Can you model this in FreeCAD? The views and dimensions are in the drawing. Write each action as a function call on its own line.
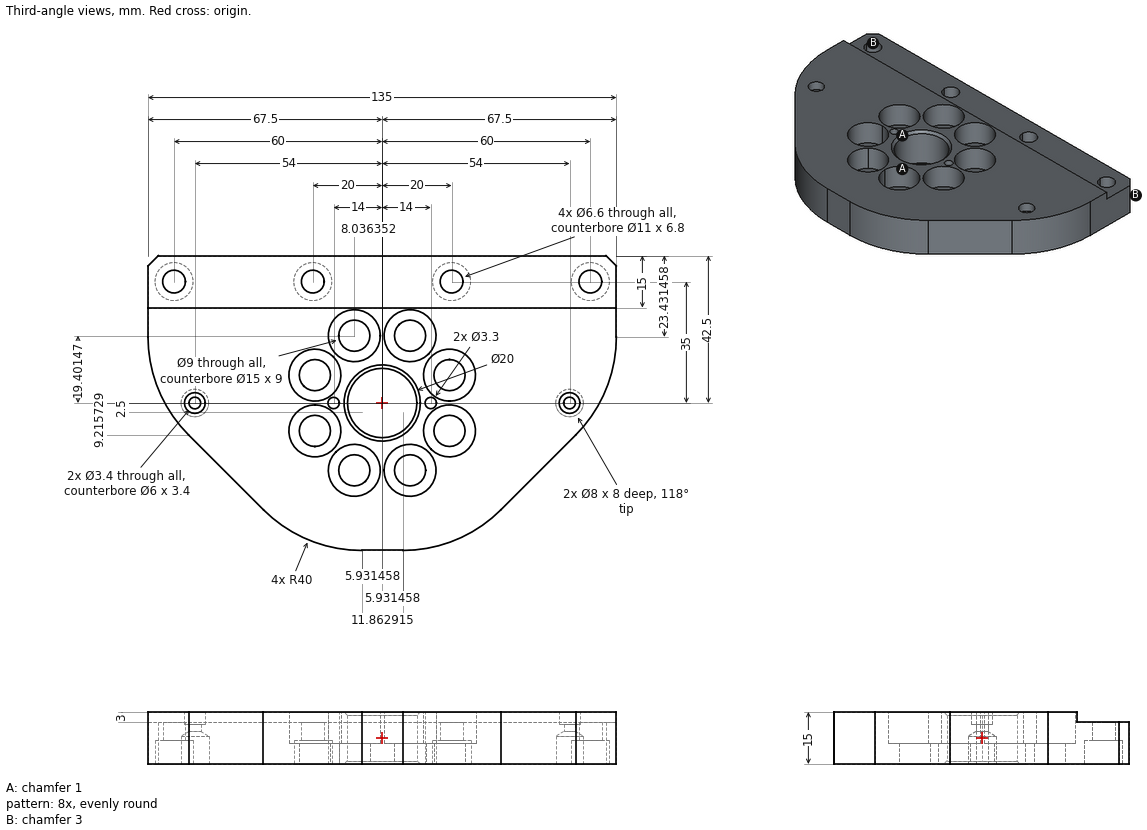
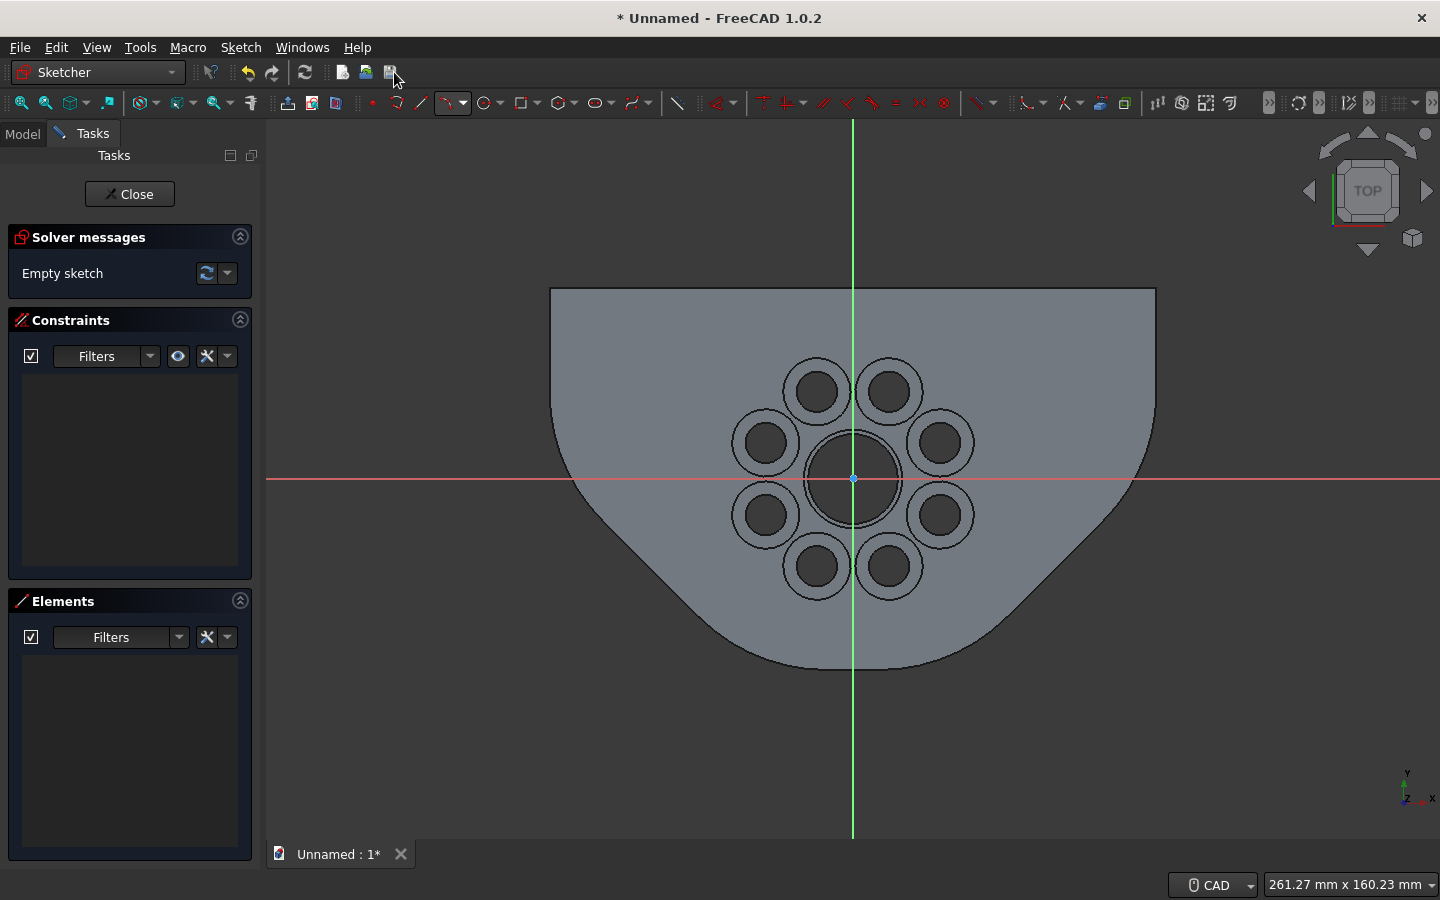
scroll(992, 479, up, 2)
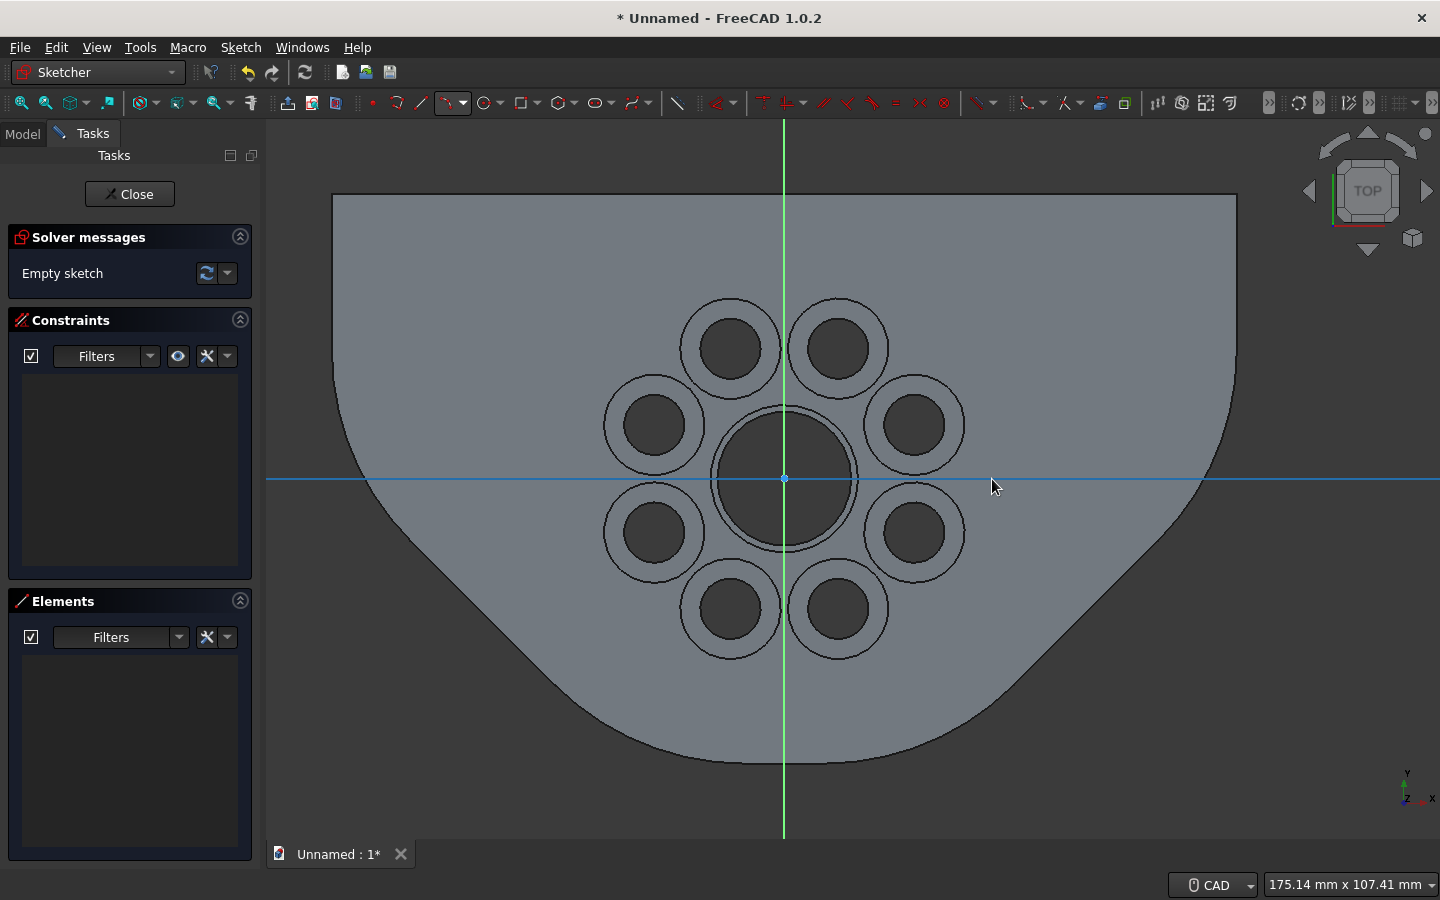
click(484, 104)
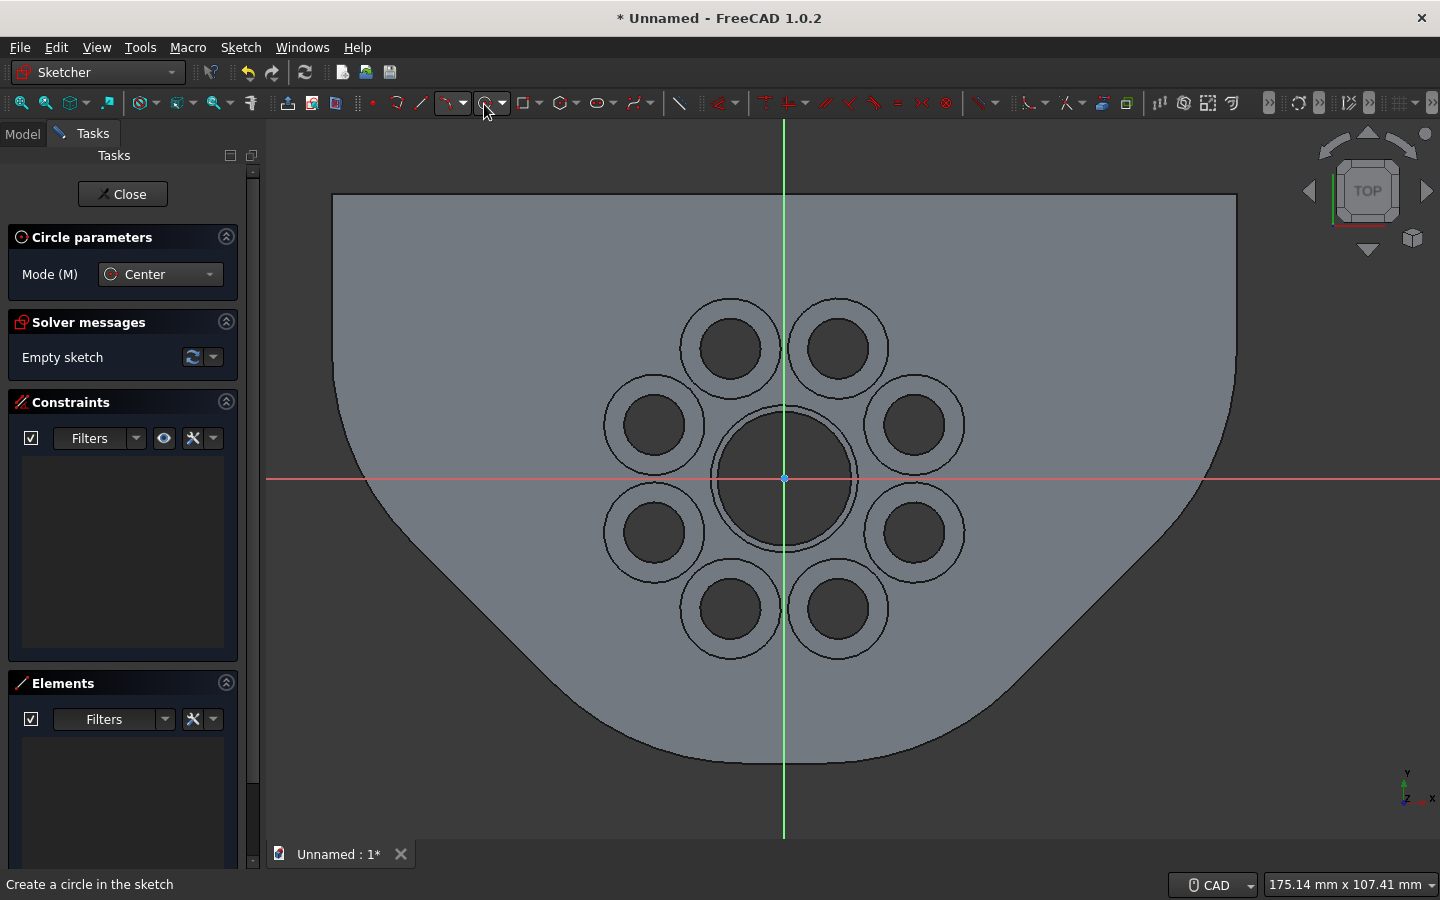
scroll(422, 479, up, 4)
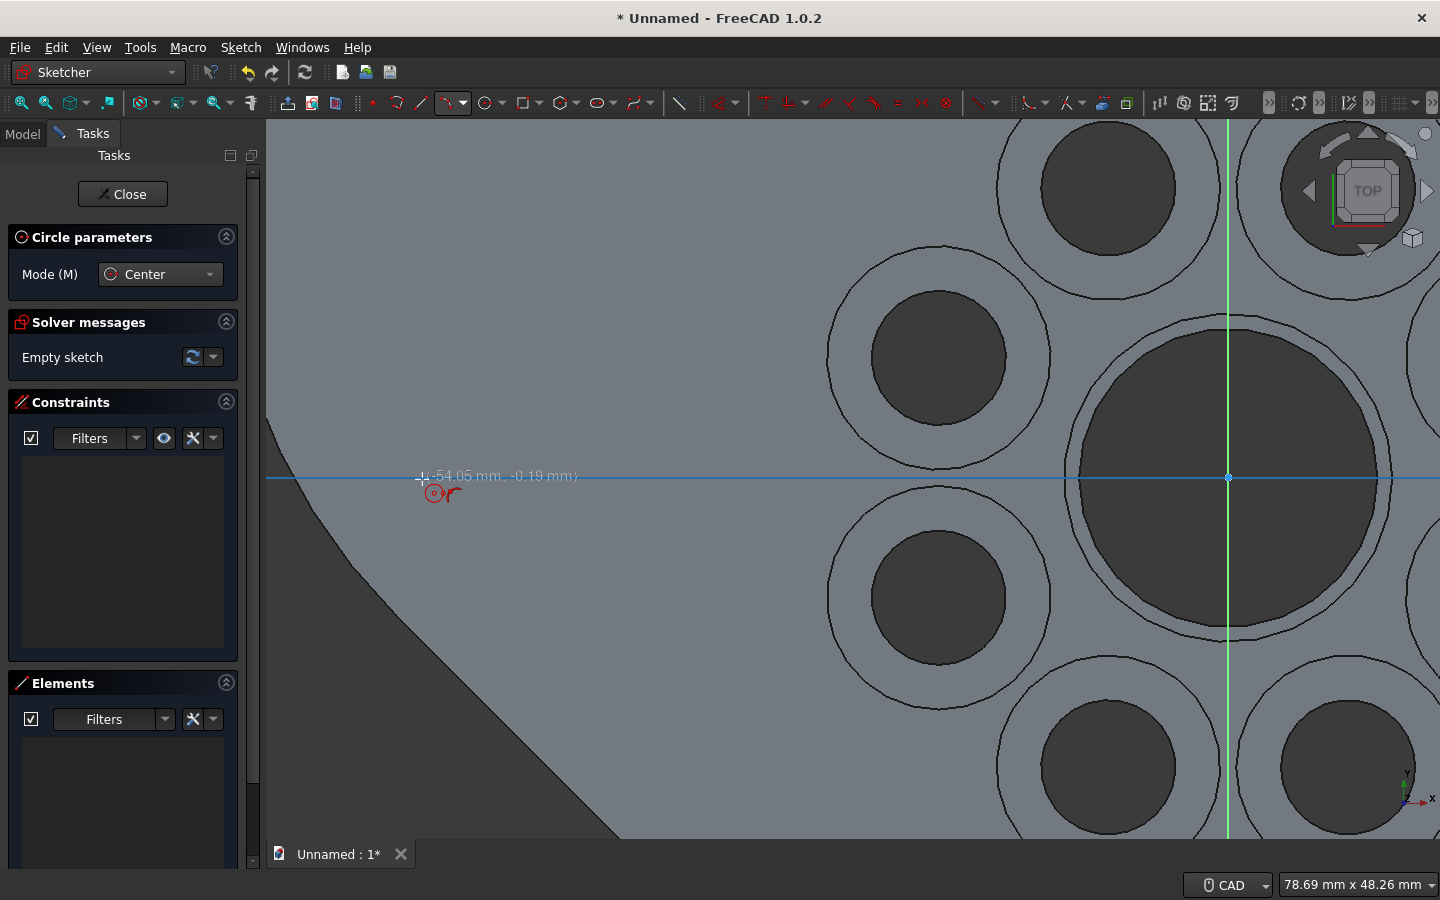
click(423, 478)
move(441, 460)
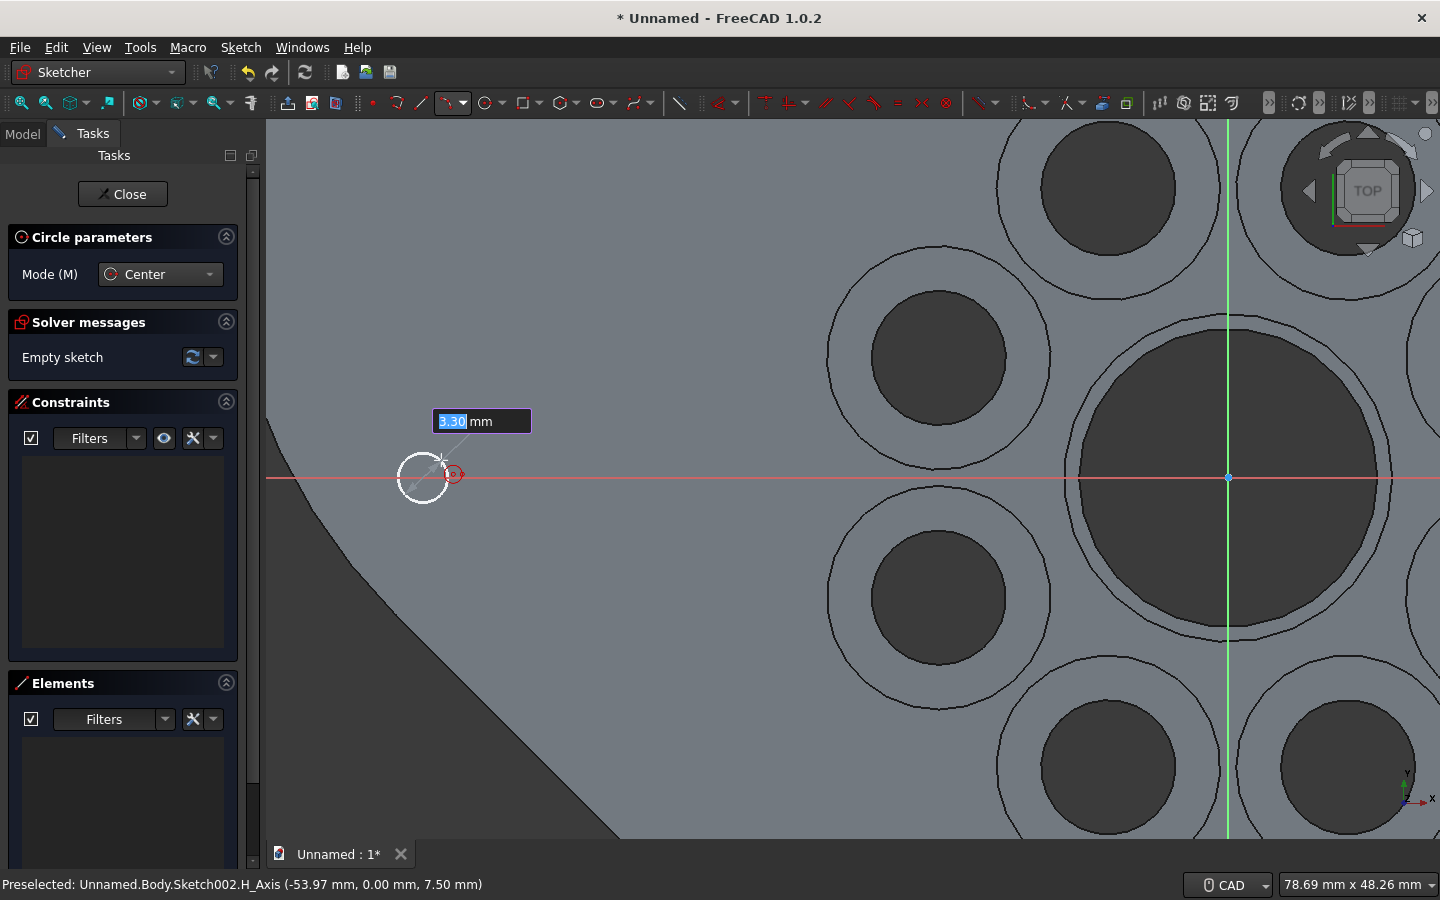
text(3.4)
key(Return)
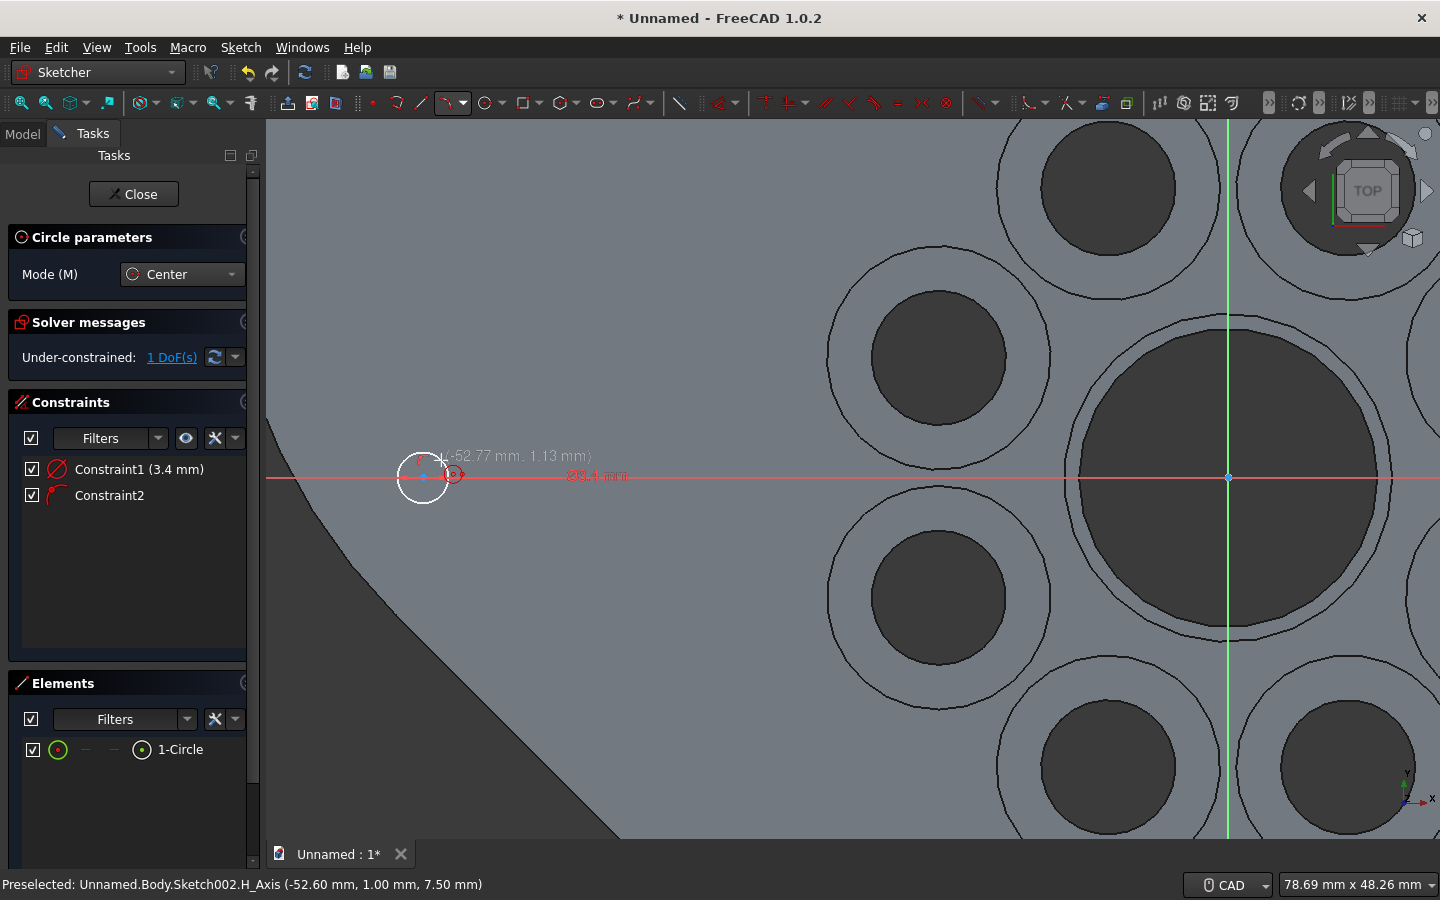
scroll(422, 480, down, 4)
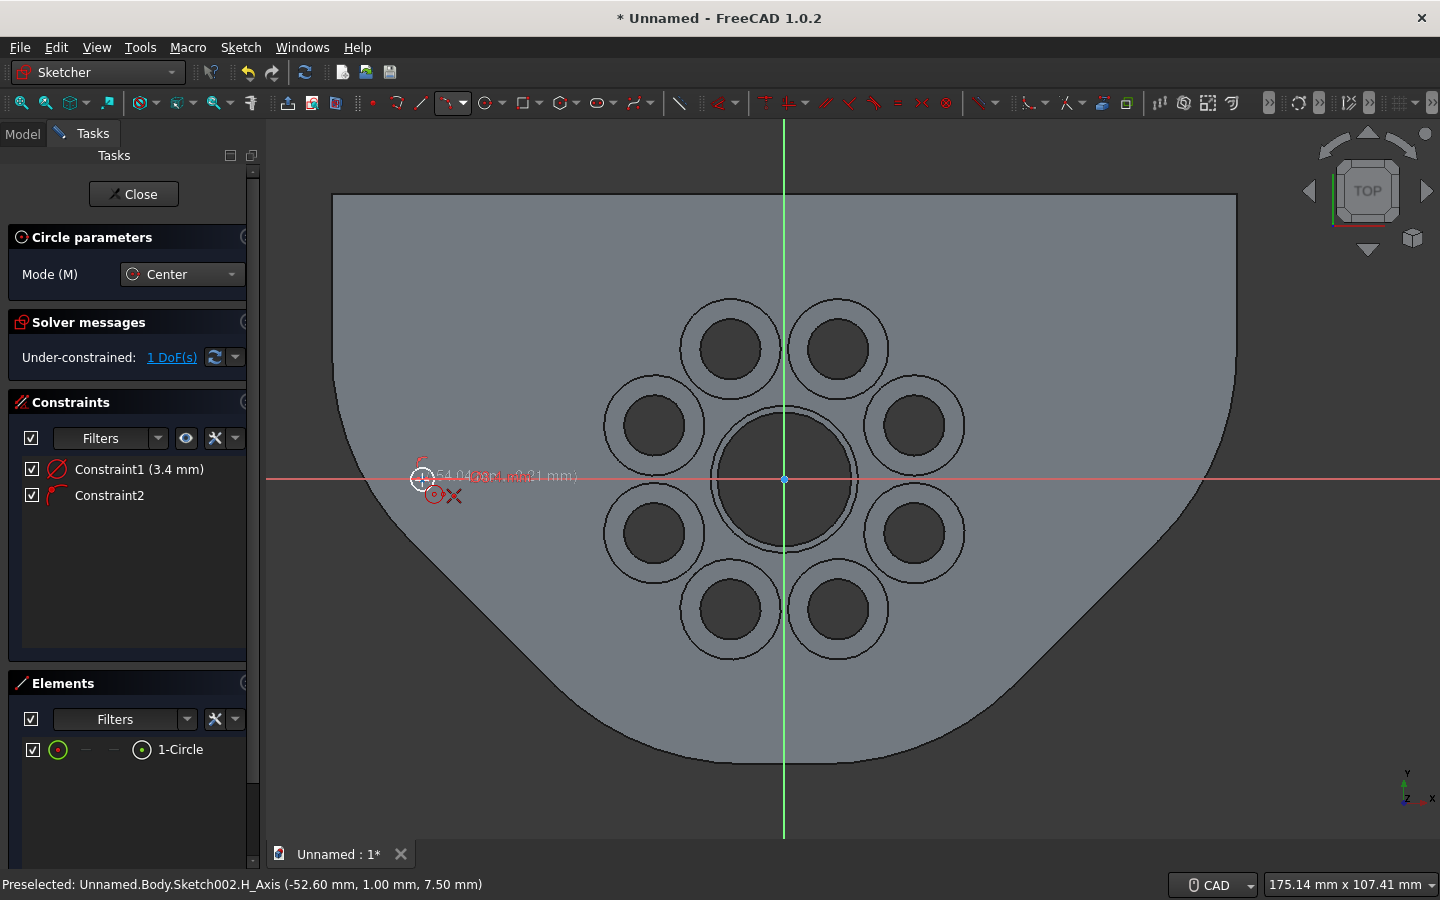
scroll(1146, 479, up, 4)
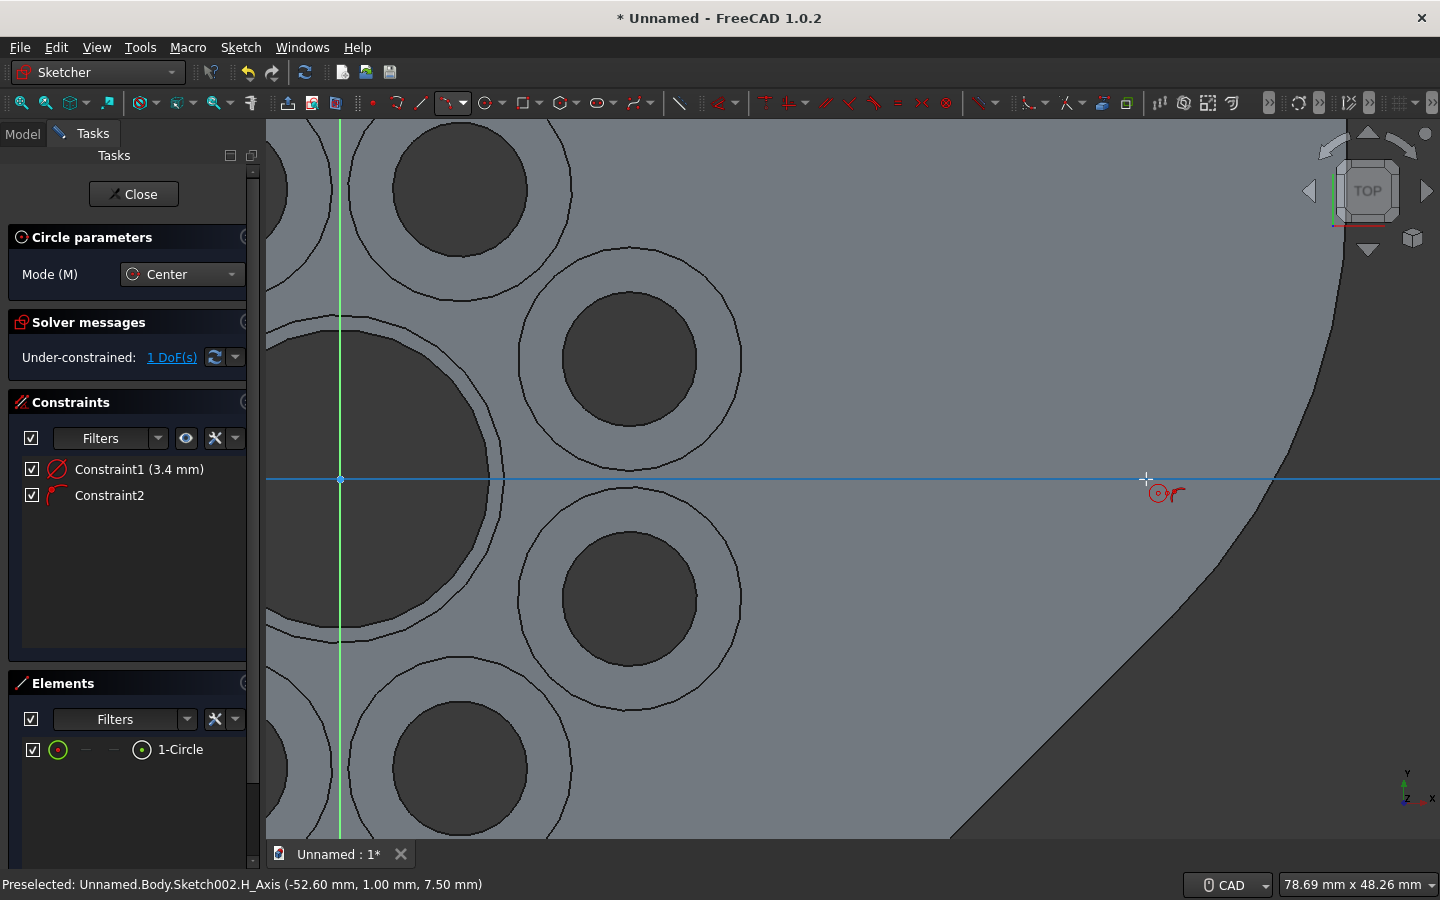
click(1146, 479)
move(1164, 461)